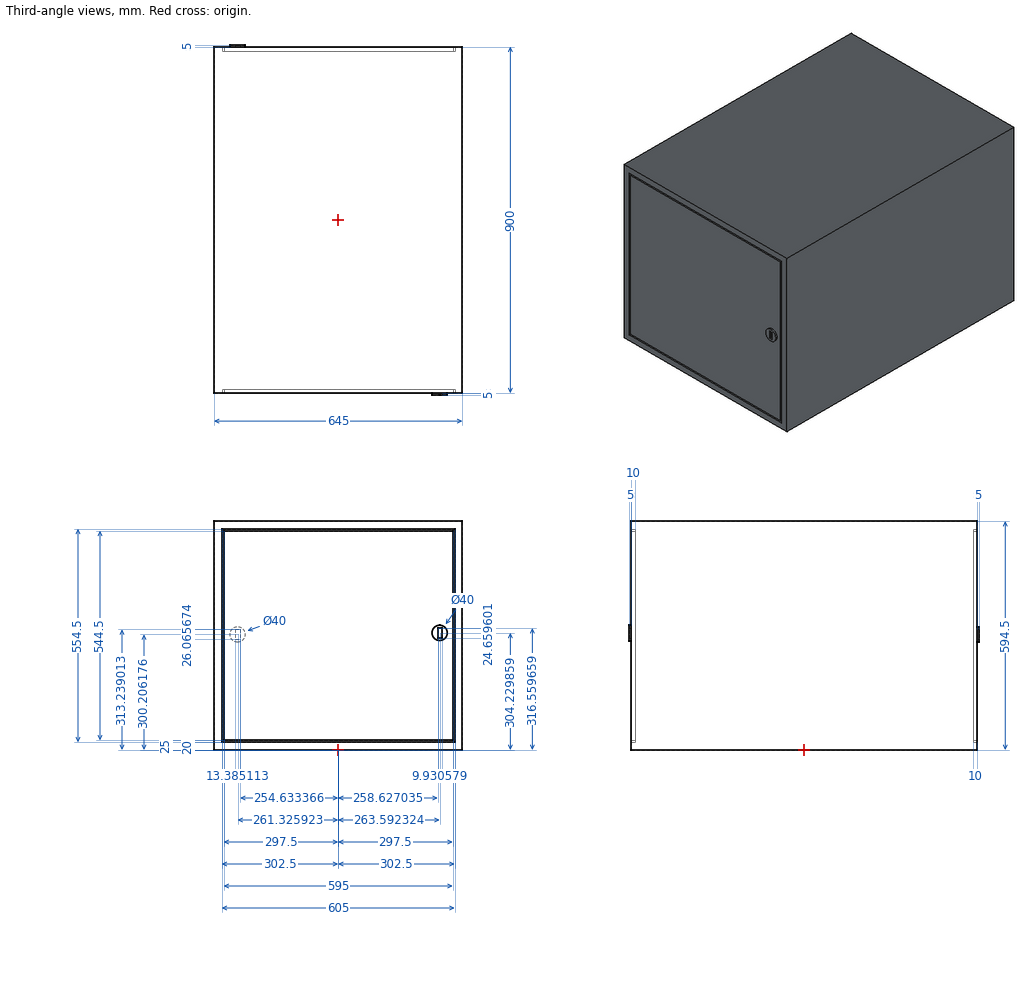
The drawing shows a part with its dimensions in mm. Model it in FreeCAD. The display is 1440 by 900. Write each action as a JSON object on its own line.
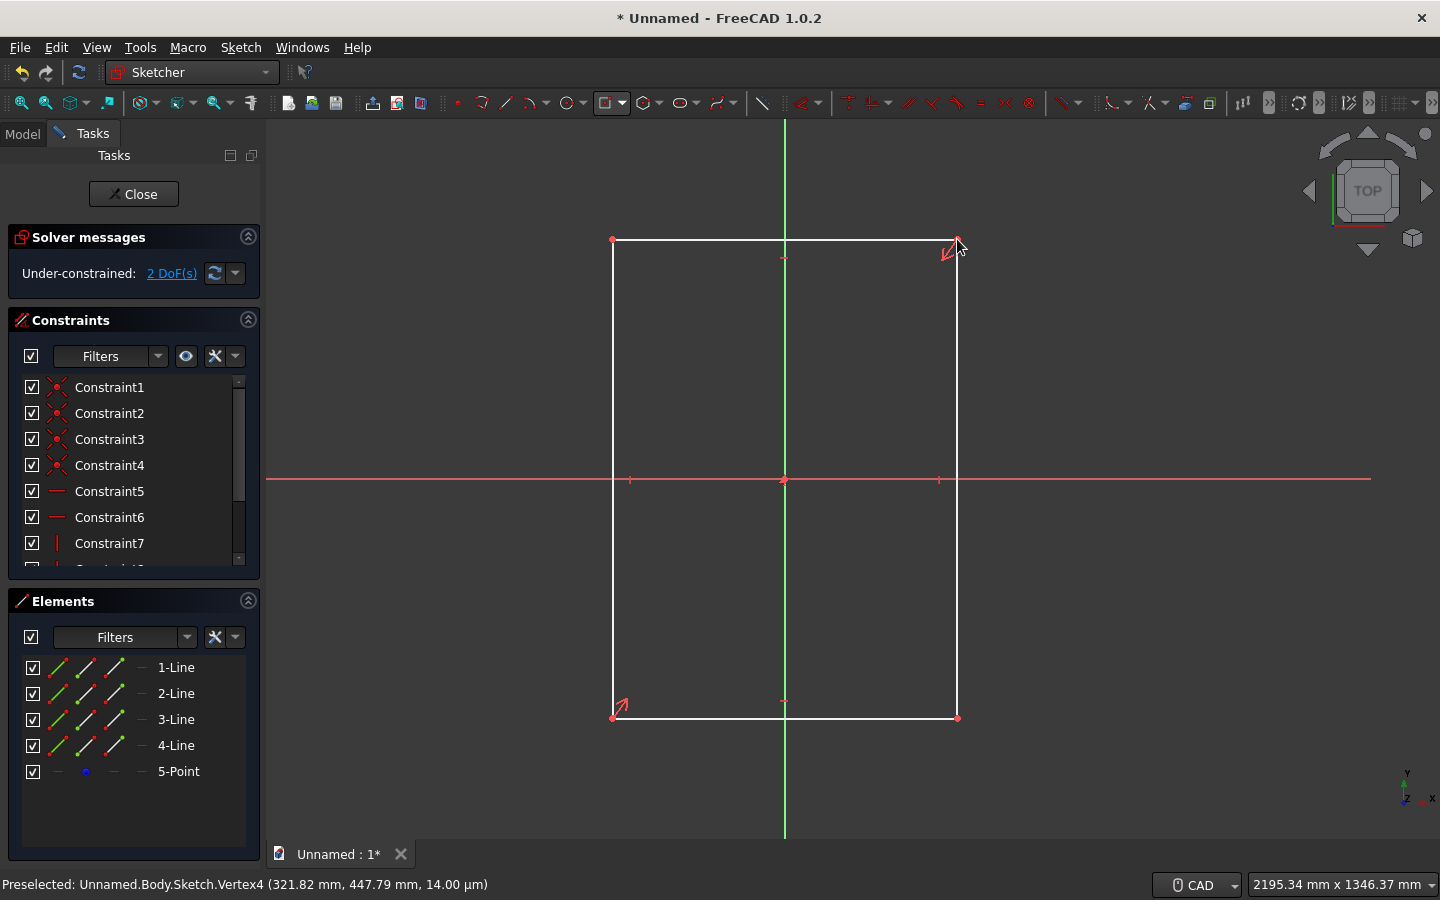
{"action": "key", "text": "d"}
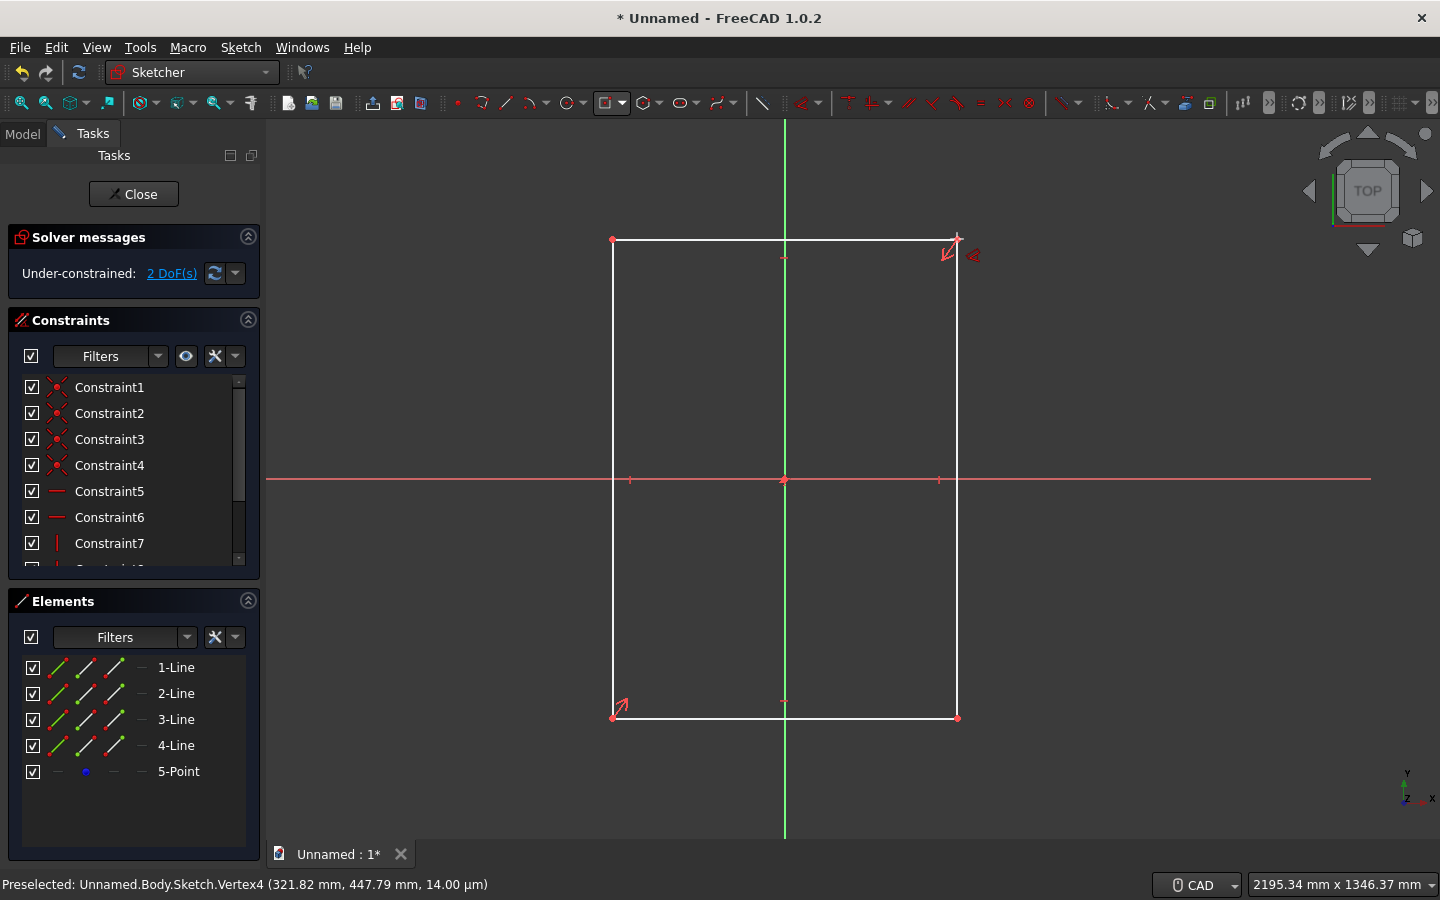
{"action": "left_click", "coordinate": [716, 719]}
{"action": "left_click", "coordinate": [706, 753]}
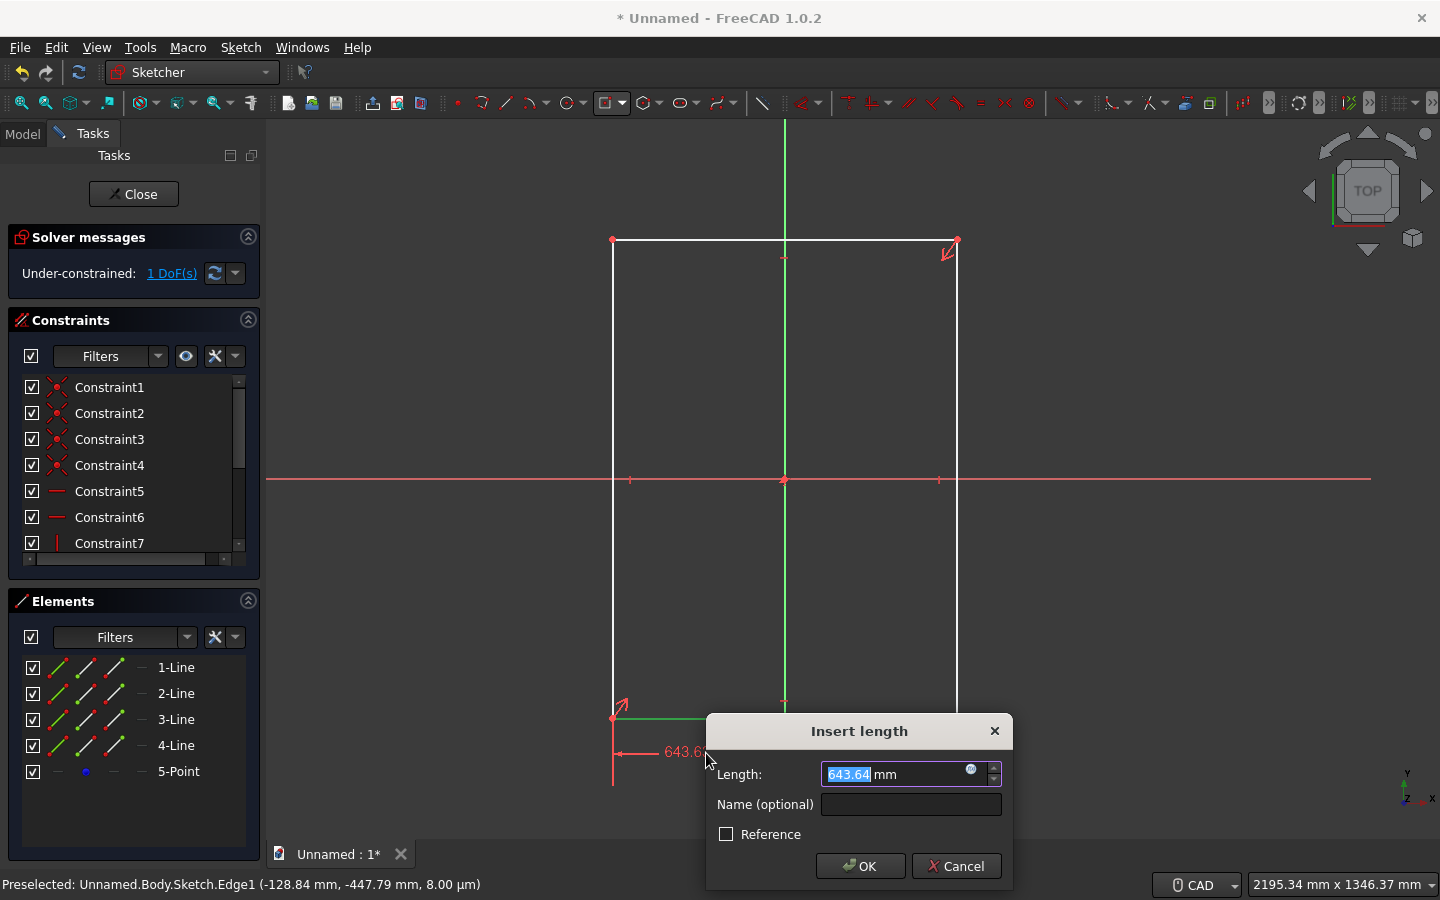
{"action": "type", "text": "645"}
{"action": "key", "text": "Return"}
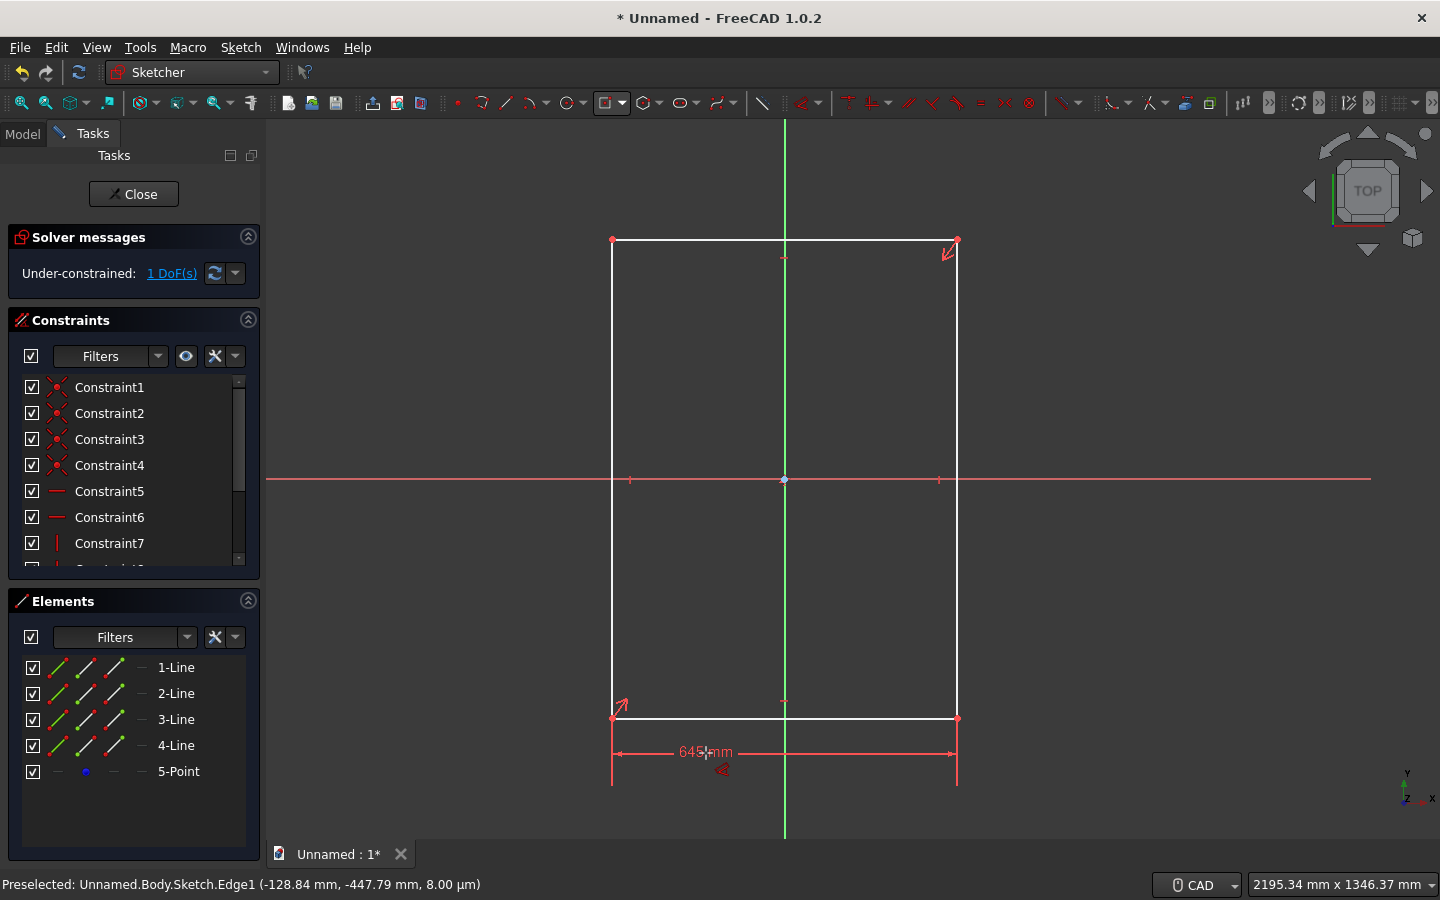
{"action": "left_click", "coordinate": [957, 575]}
{"action": "left_click", "coordinate": [991, 369]}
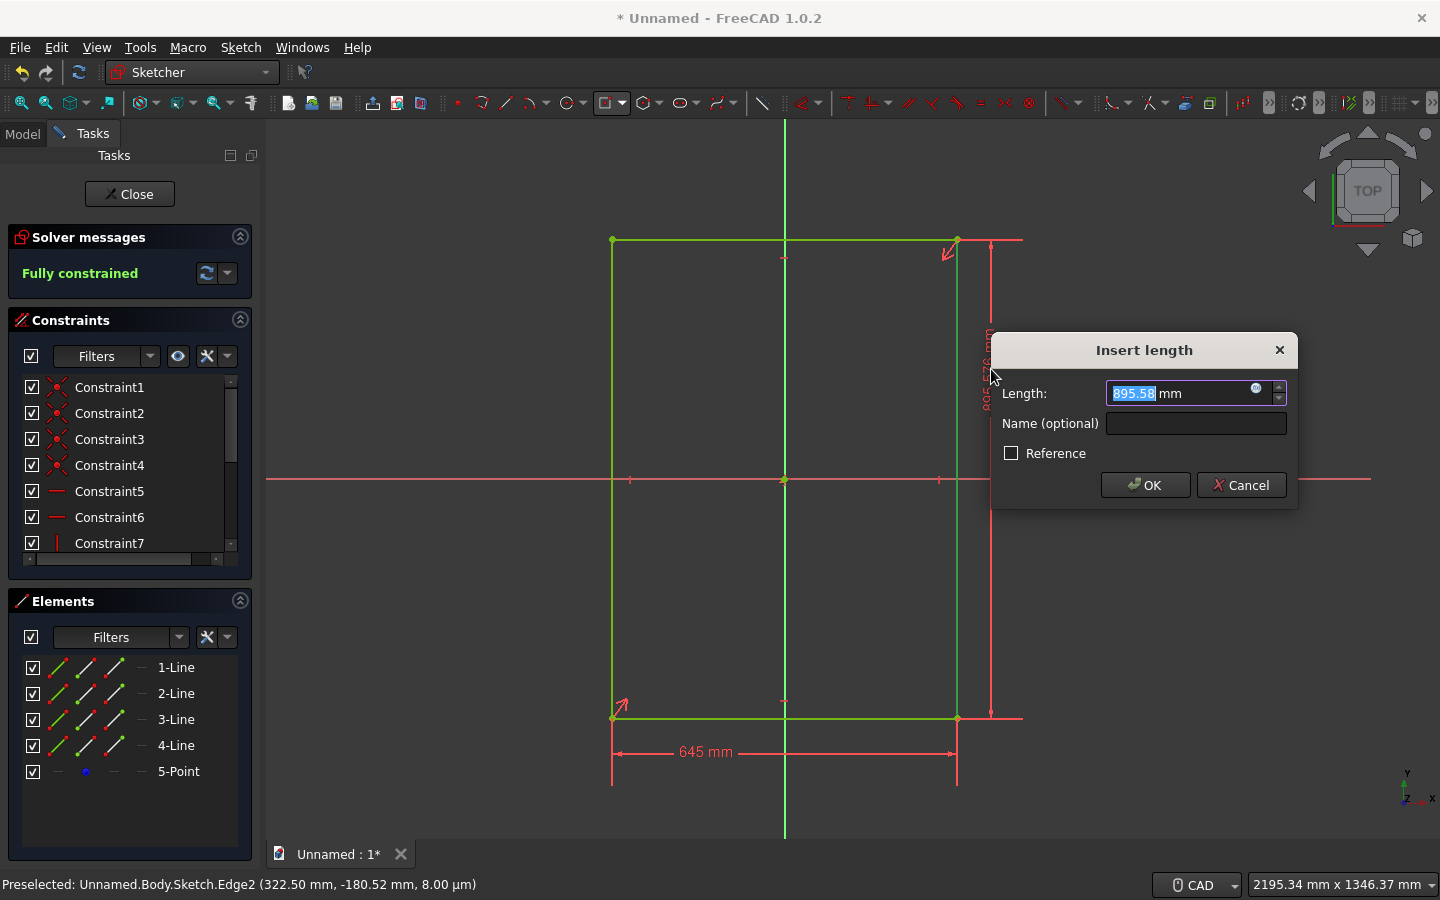
{"action": "type", "text": "900"}
{"action": "key", "text": "Return"}
{"action": "key", "text": "Escape"}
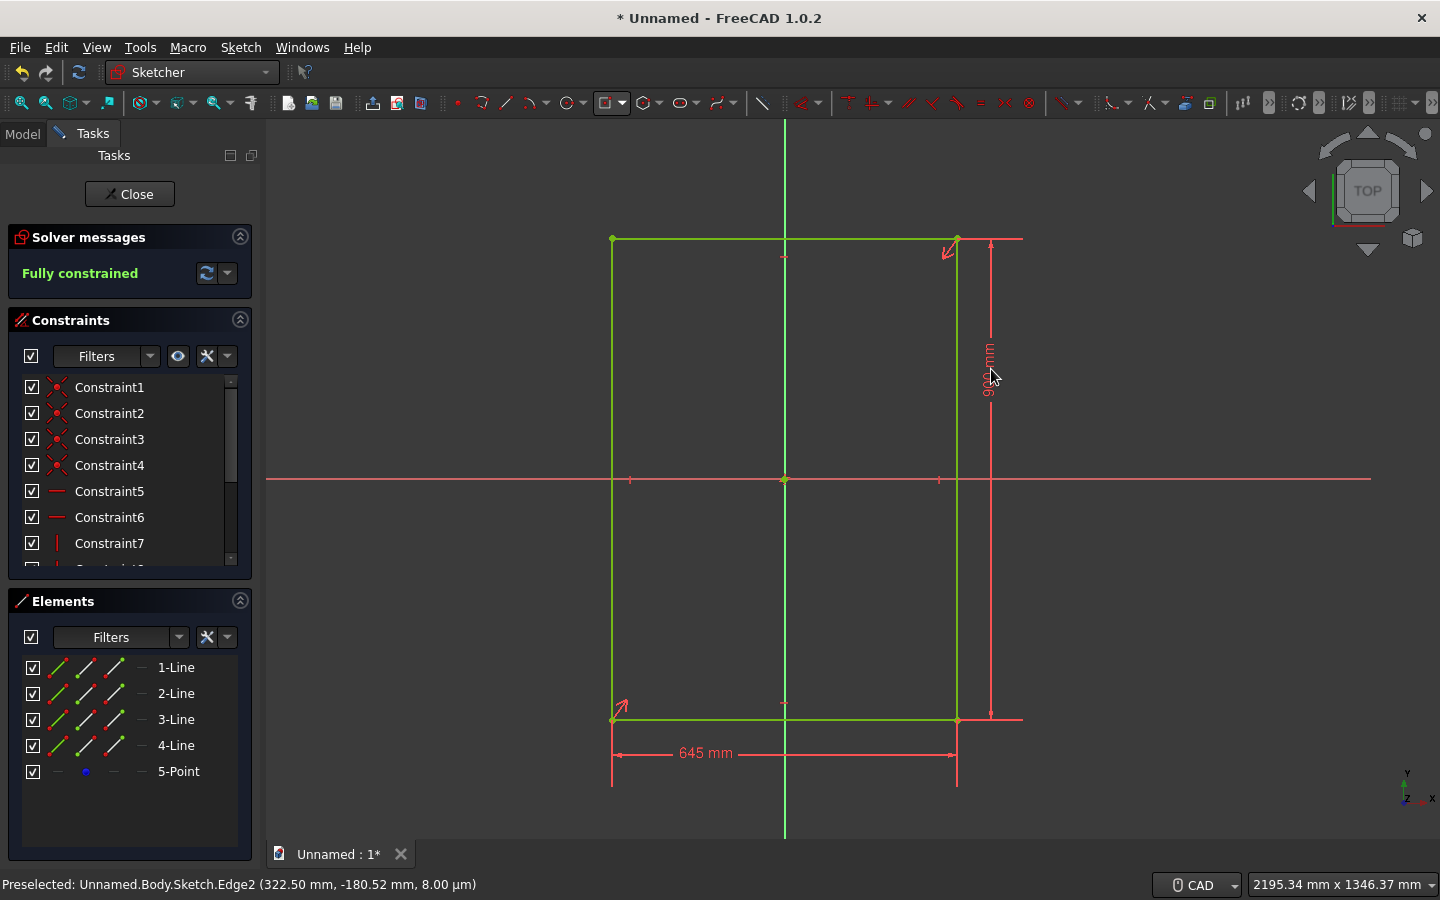
{"action": "left_click", "coordinate": [130, 194]}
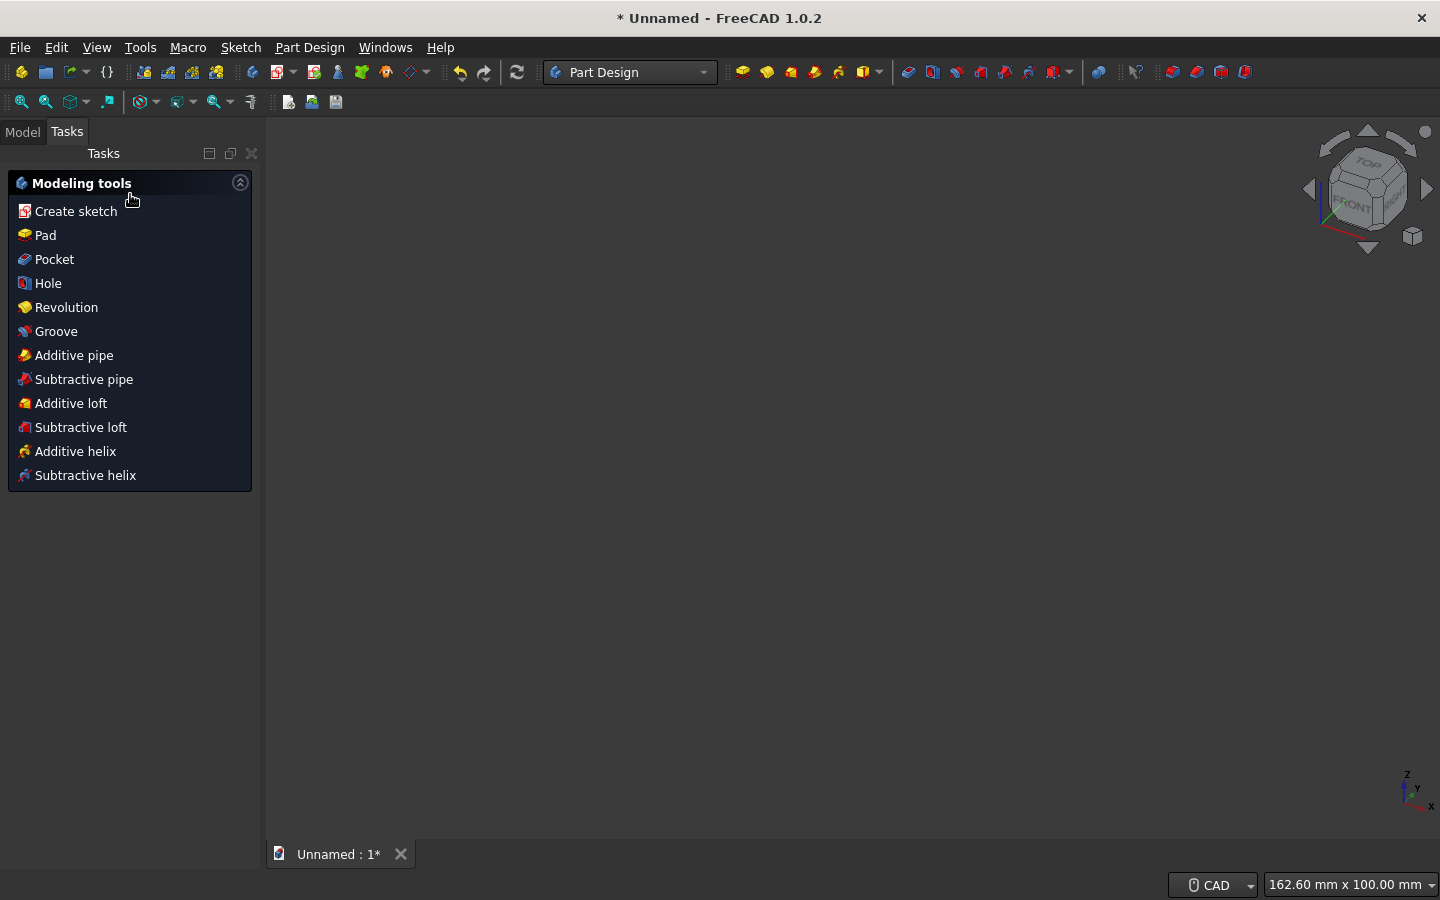
{"action": "left_click", "coordinate": [744, 72]}